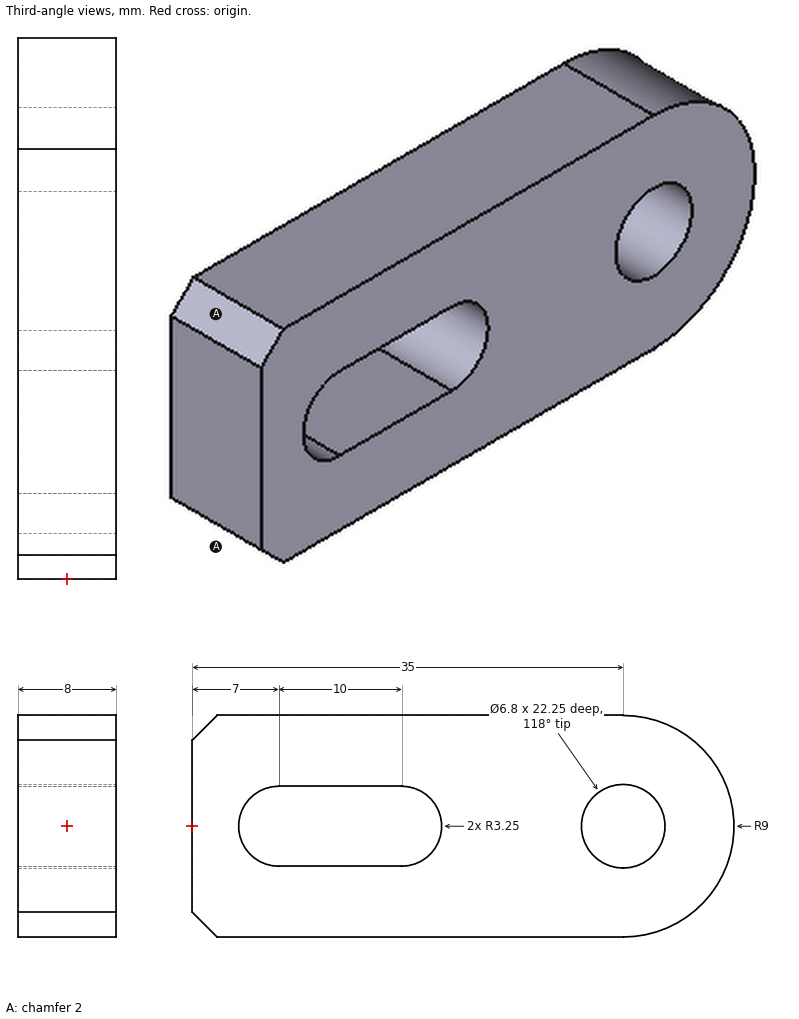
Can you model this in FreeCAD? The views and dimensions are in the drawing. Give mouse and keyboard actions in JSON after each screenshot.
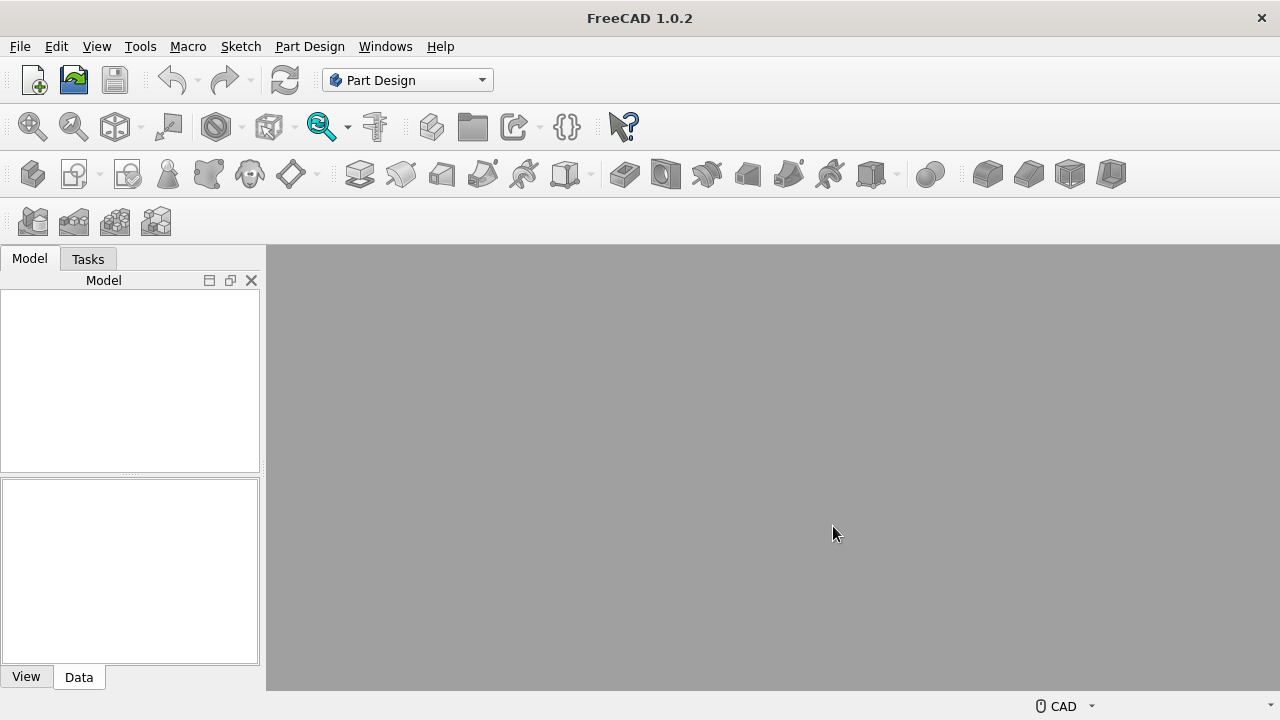
{"action": "left_click", "coordinate": [33, 80]}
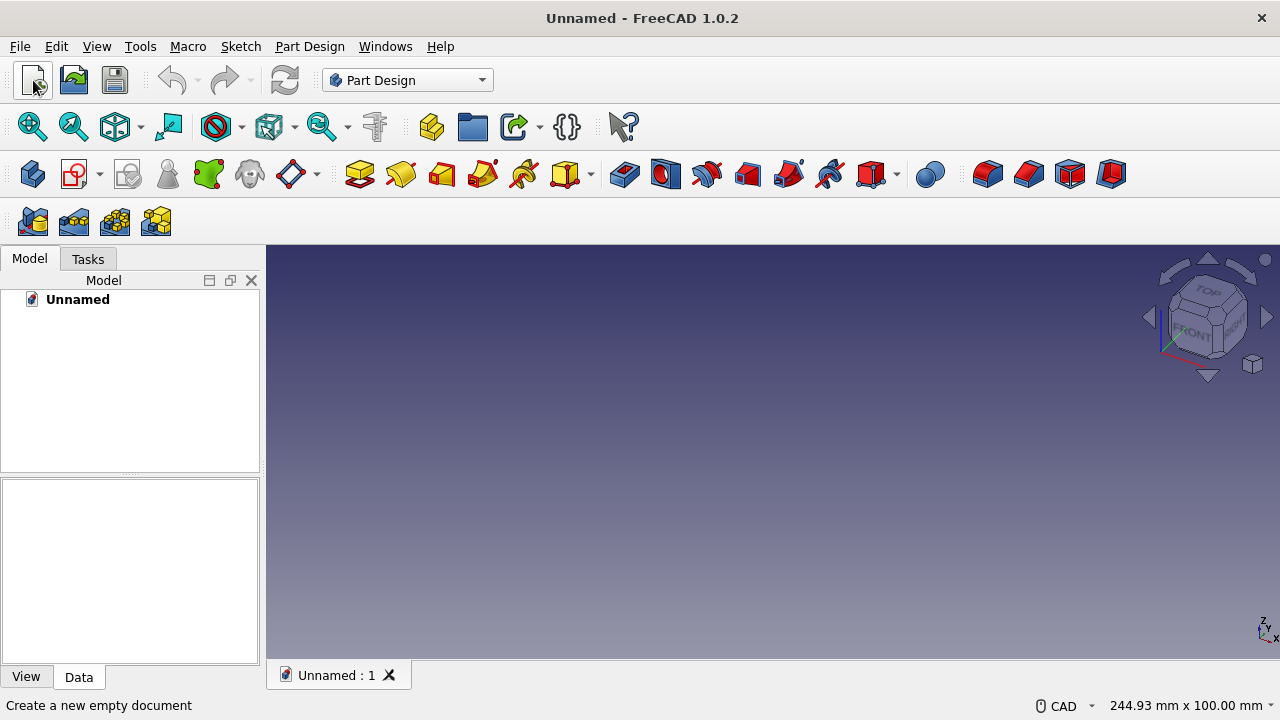
{"action": "left_click", "coordinate": [74, 174]}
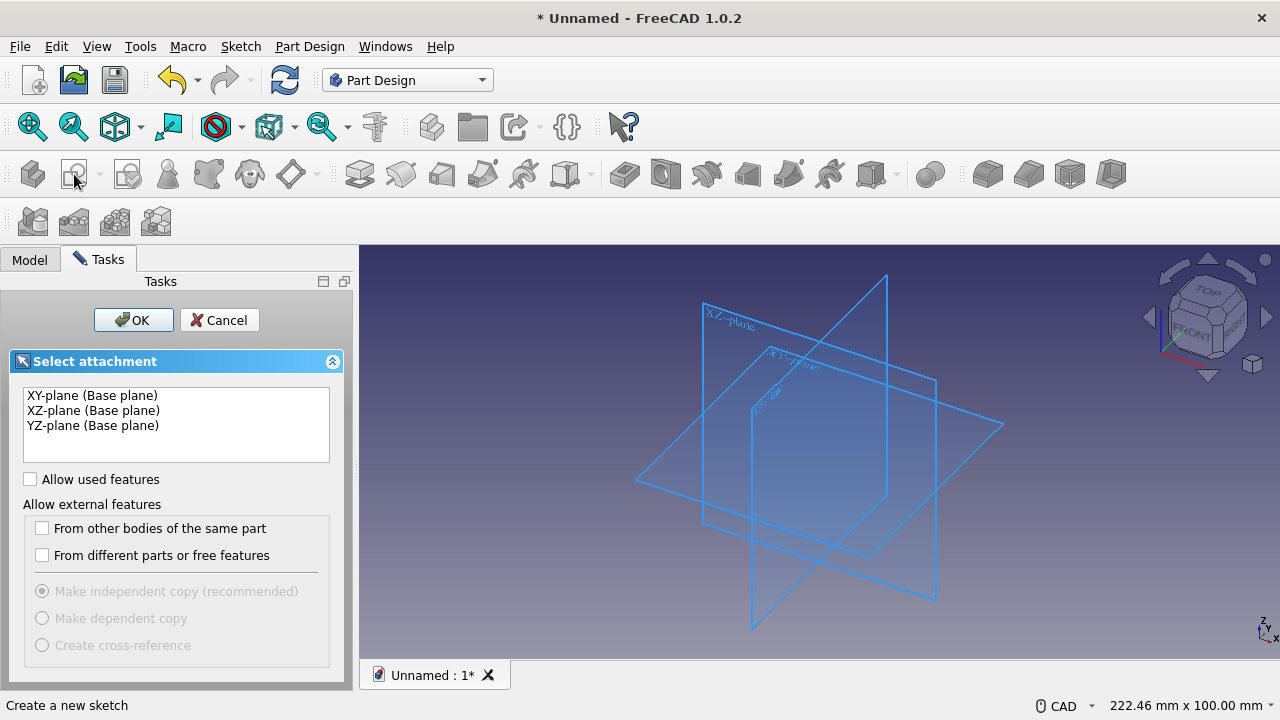
{"action": "left_click", "coordinate": [84, 426]}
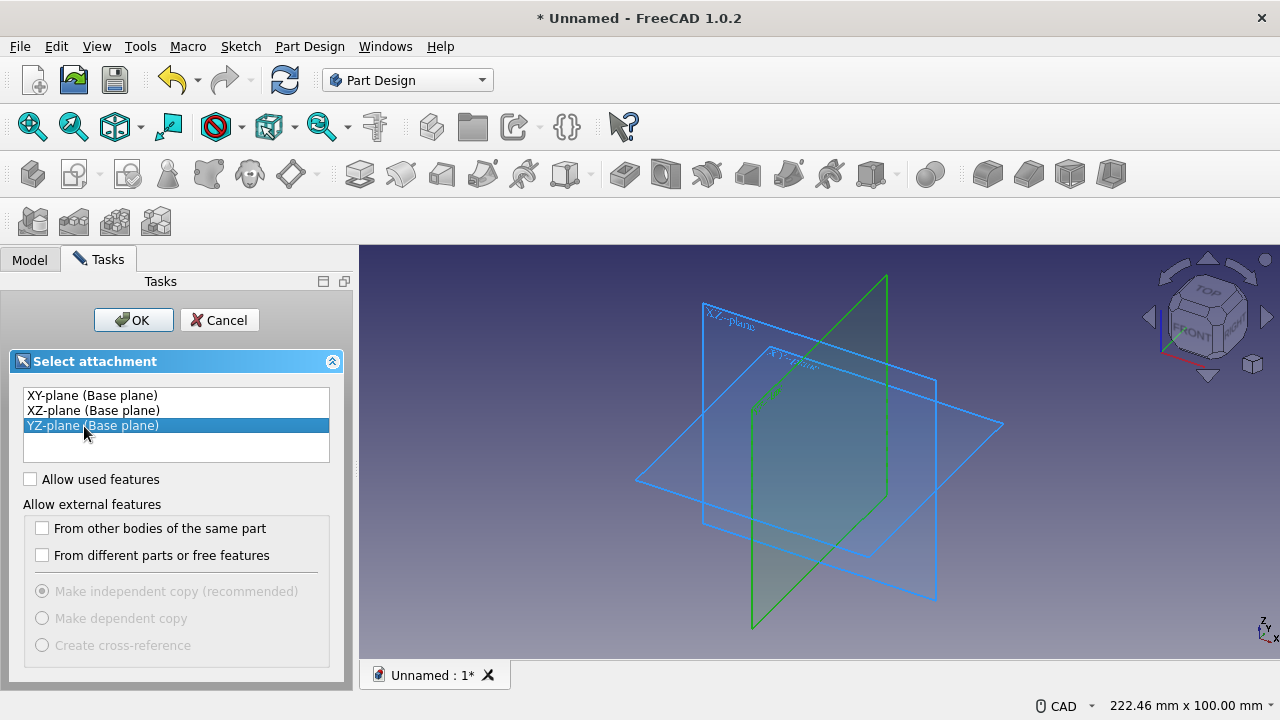
{"action": "left_click", "coordinate": [134, 320]}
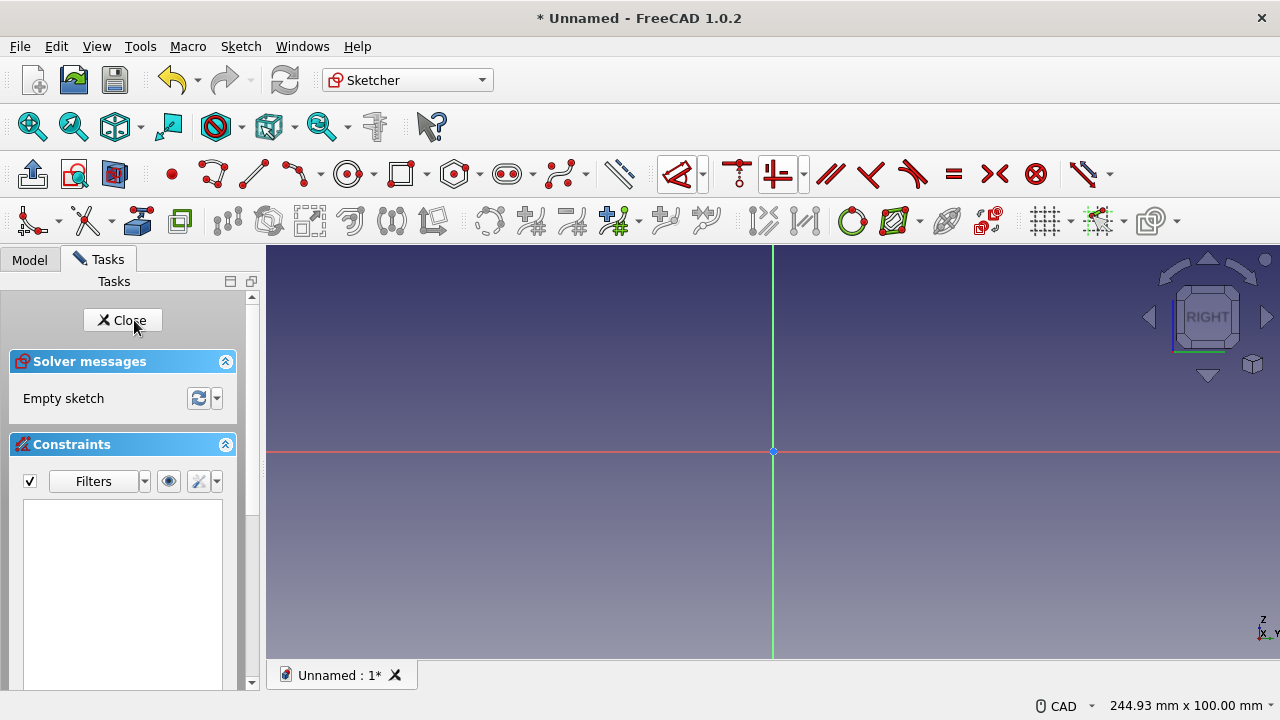
{"action": "scroll", "coordinate": [933, 452], "scroll_direction": "up", "scroll_amount": 6}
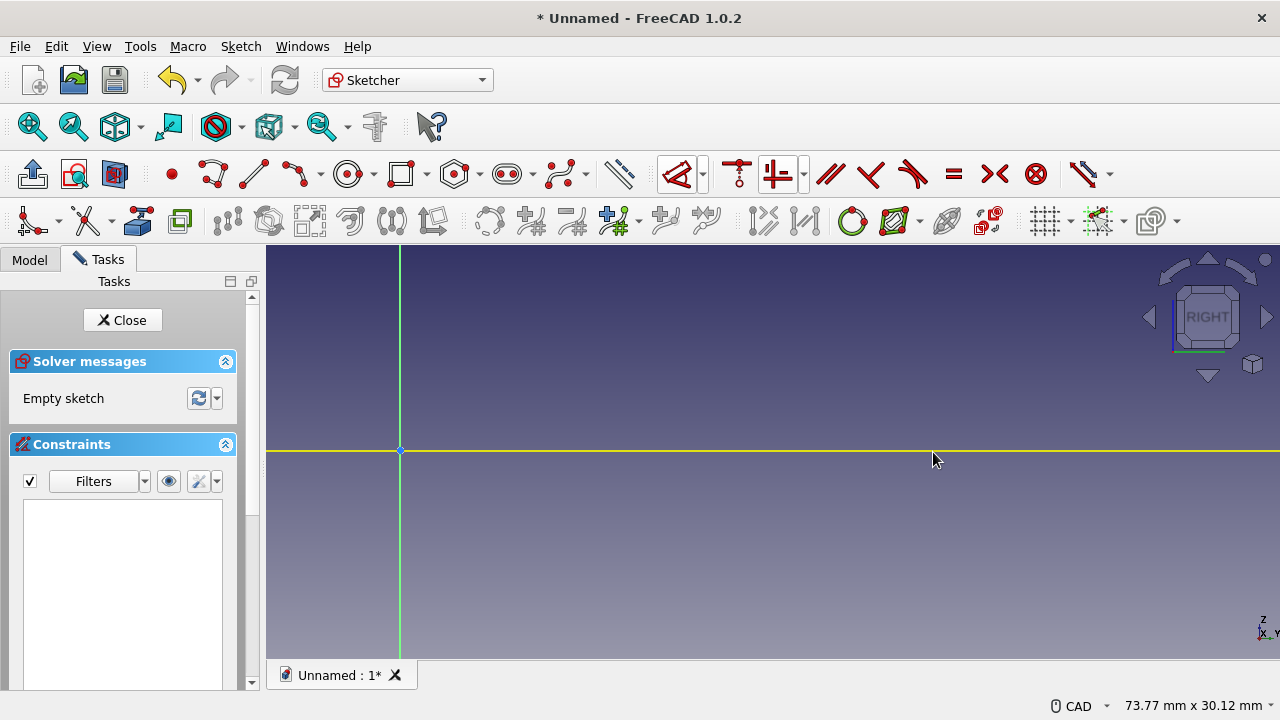
{"action": "key", "text": "g m"}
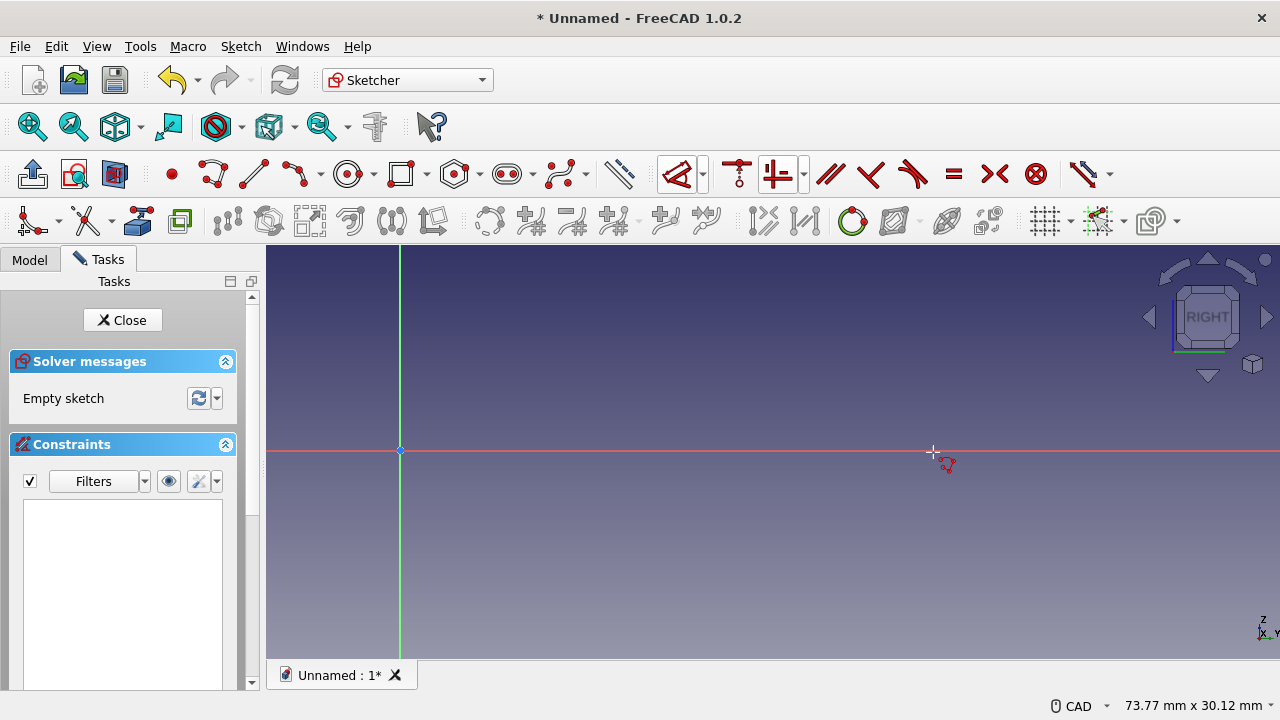
{"action": "left_click", "coordinate": [881, 327]}
{"action": "left_click", "coordinate": [400, 327]}
{"action": "left_click", "coordinate": [409, 575]}
{"action": "left_click", "coordinate": [881, 575]}
{"action": "right_click", "coordinate": [881, 575]}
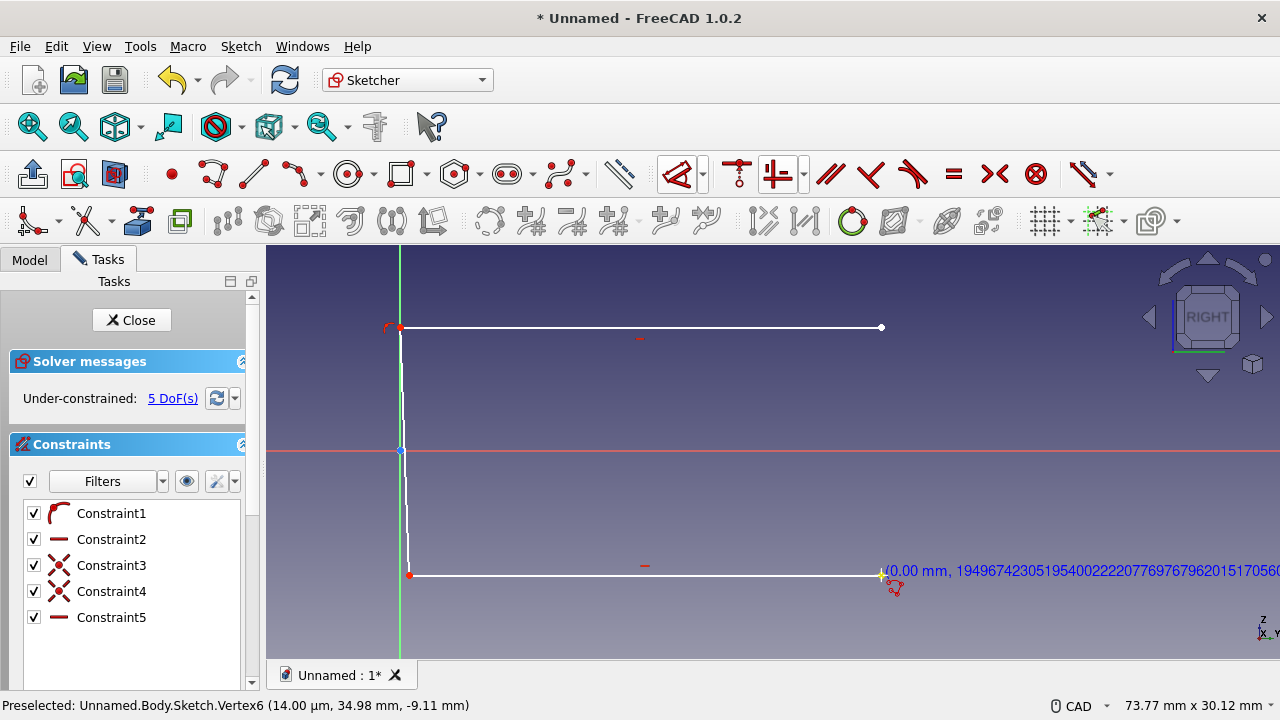
{"action": "key", "text": "g 3 a"}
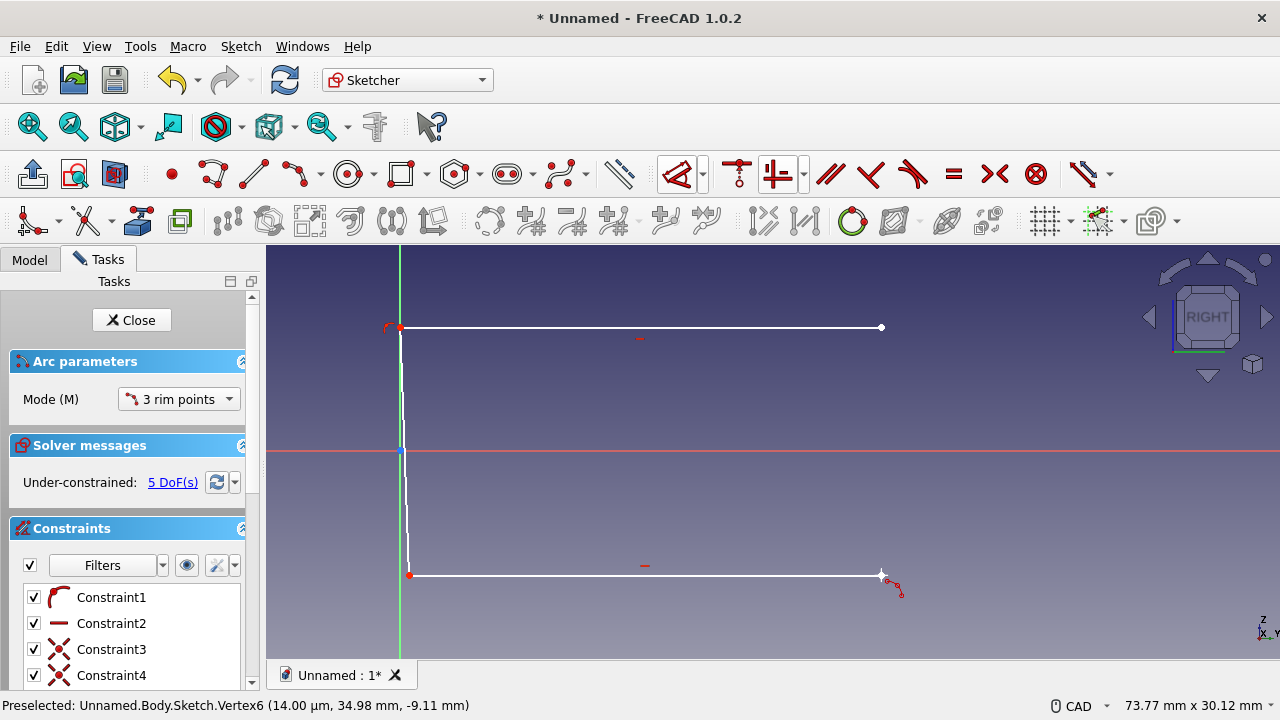
{"action": "left_click", "coordinate": [881, 576]}
{"action": "left_click", "coordinate": [881, 328]}
{"action": "left_click", "coordinate": [999, 489]}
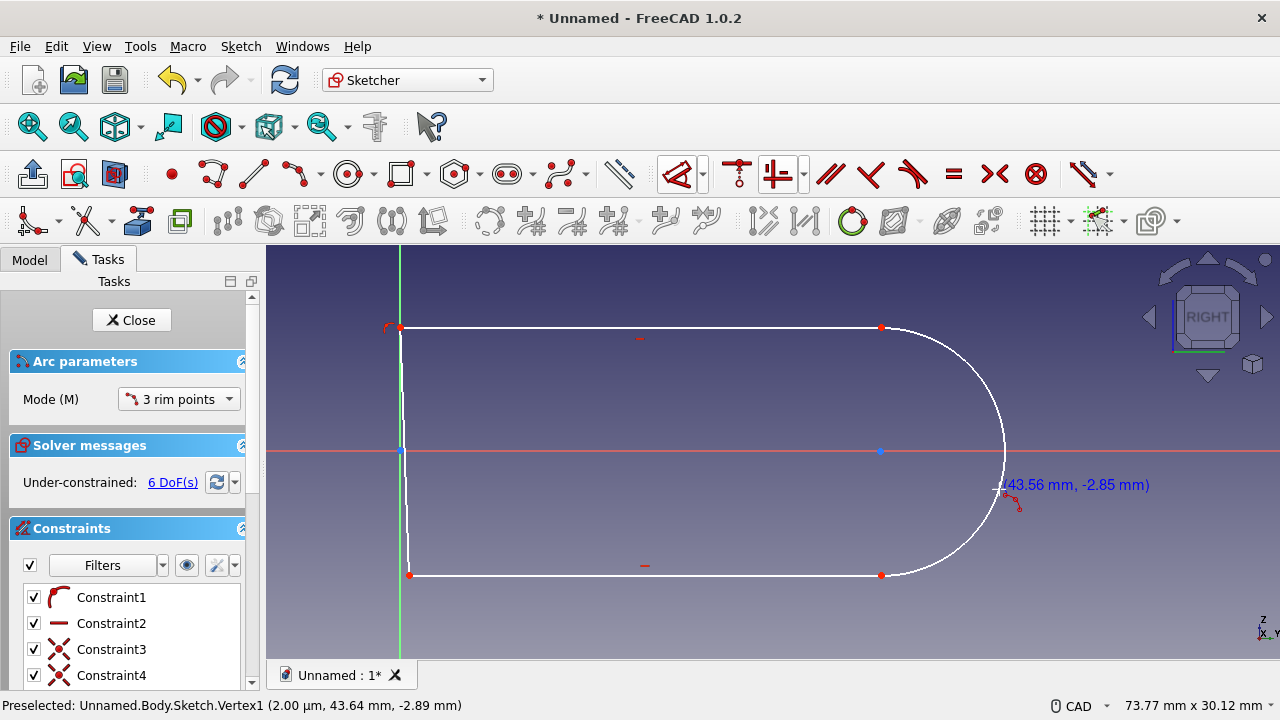
{"action": "key", "text": "g s"}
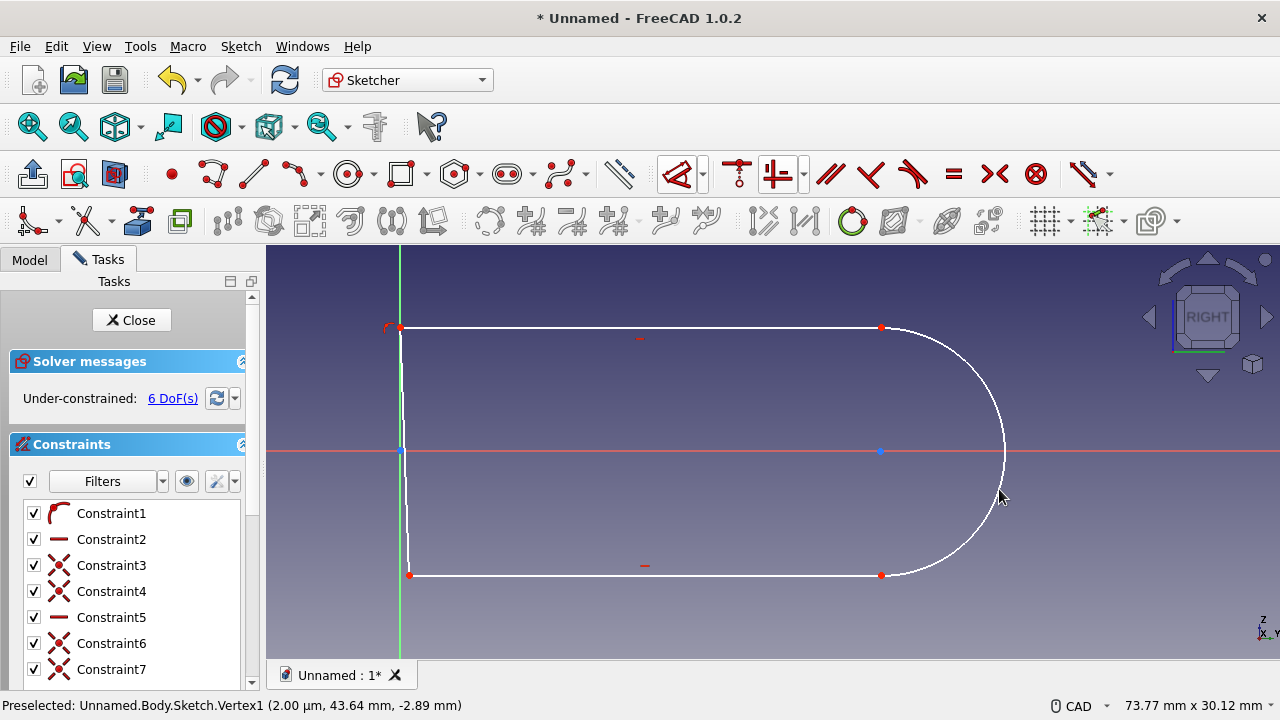
{"action": "left_click", "coordinate": [496, 451]}